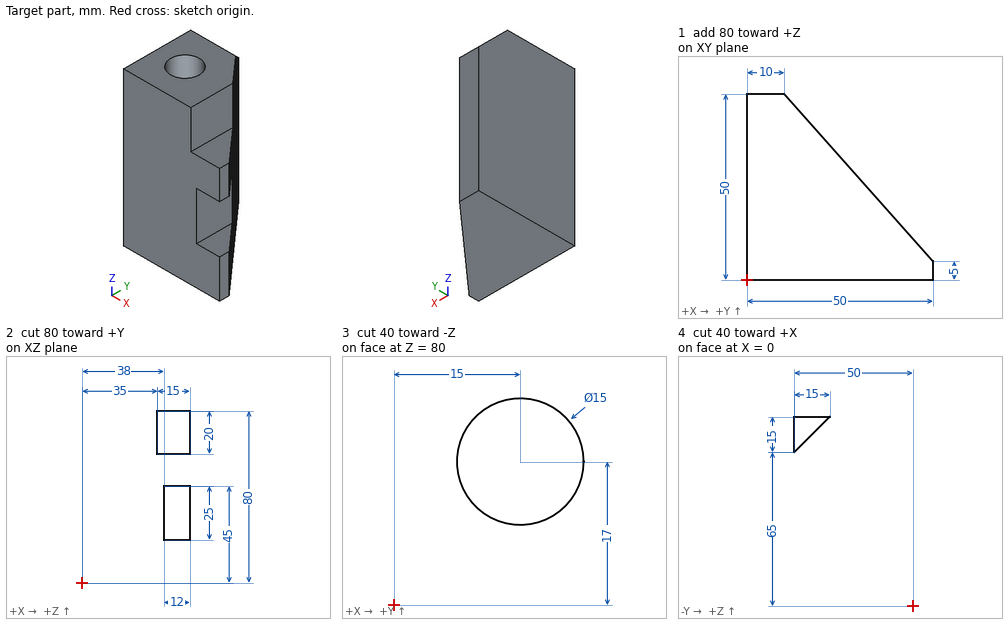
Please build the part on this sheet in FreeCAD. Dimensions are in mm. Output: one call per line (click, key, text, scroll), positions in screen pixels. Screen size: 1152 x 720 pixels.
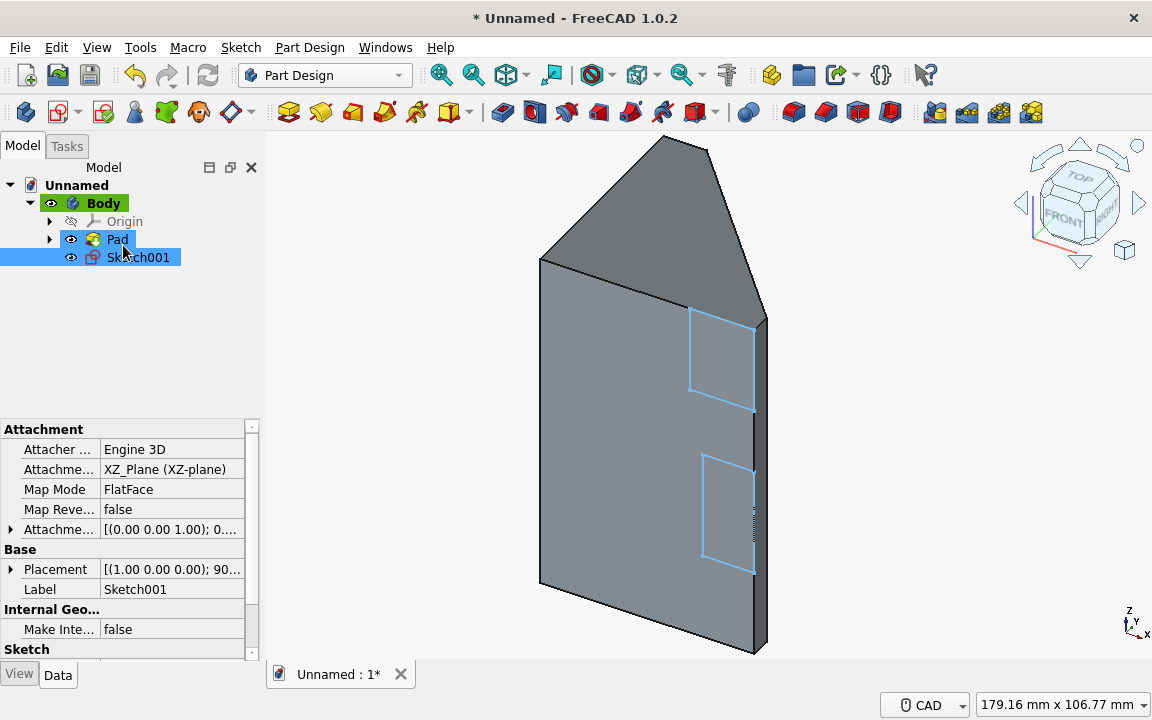
click(504, 112)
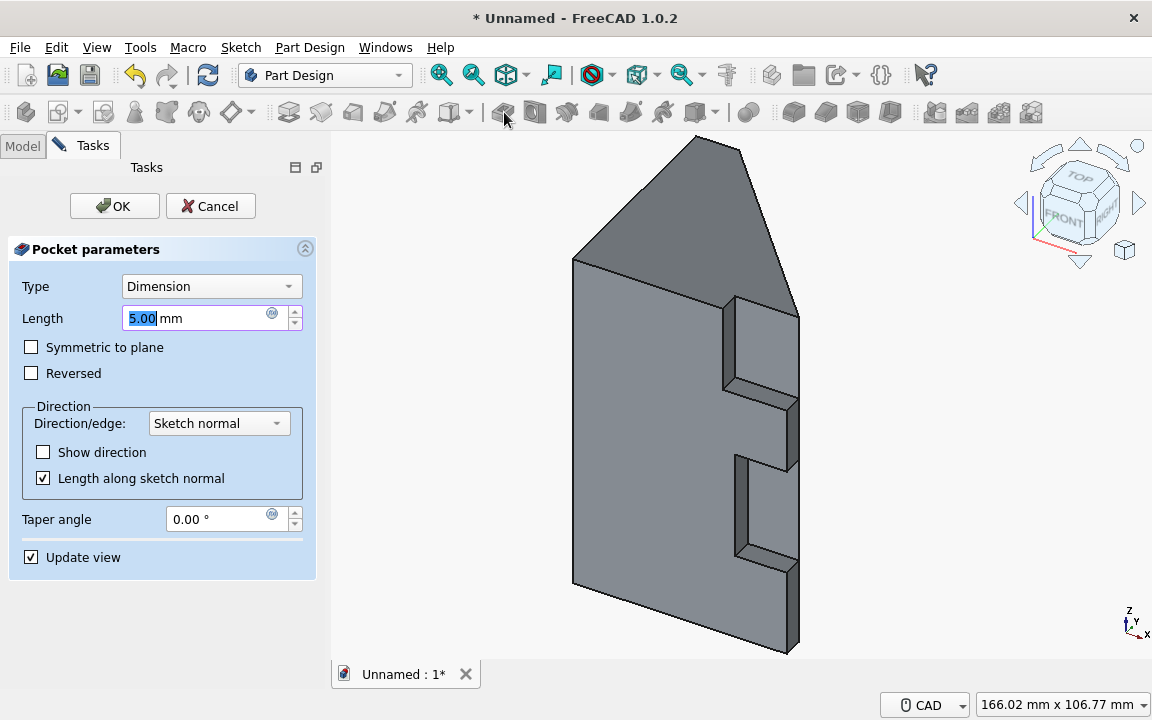
text(80)
key(Tab)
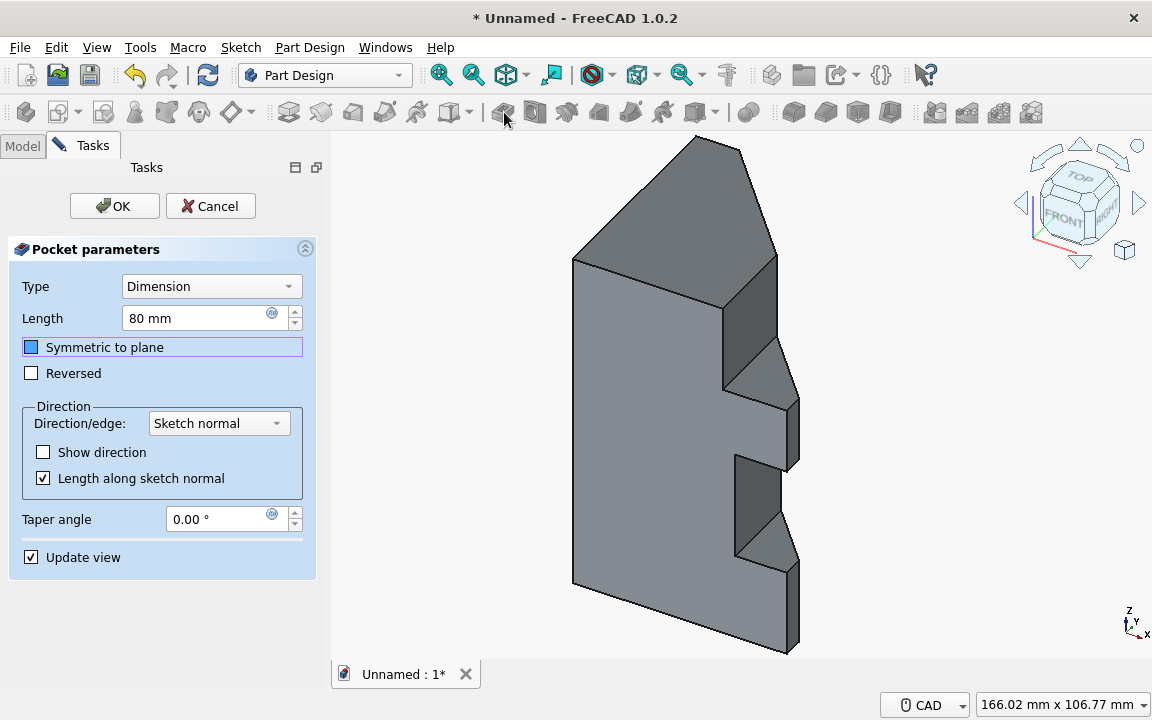
click(115, 206)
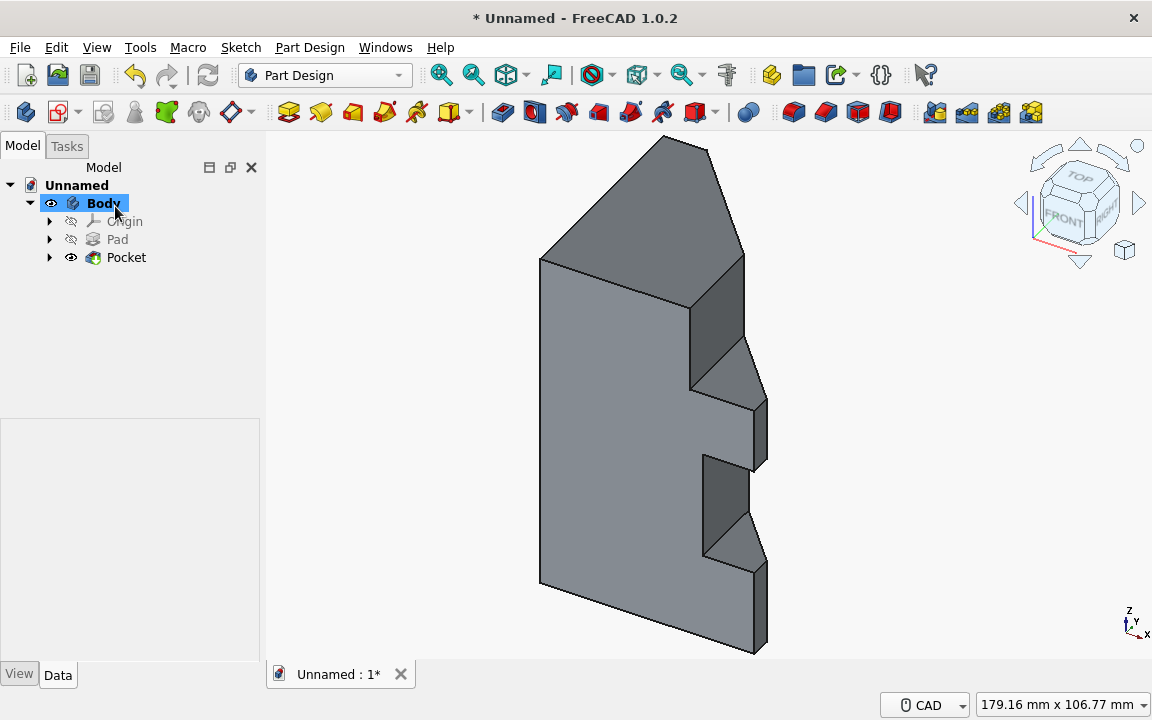
click(659, 239)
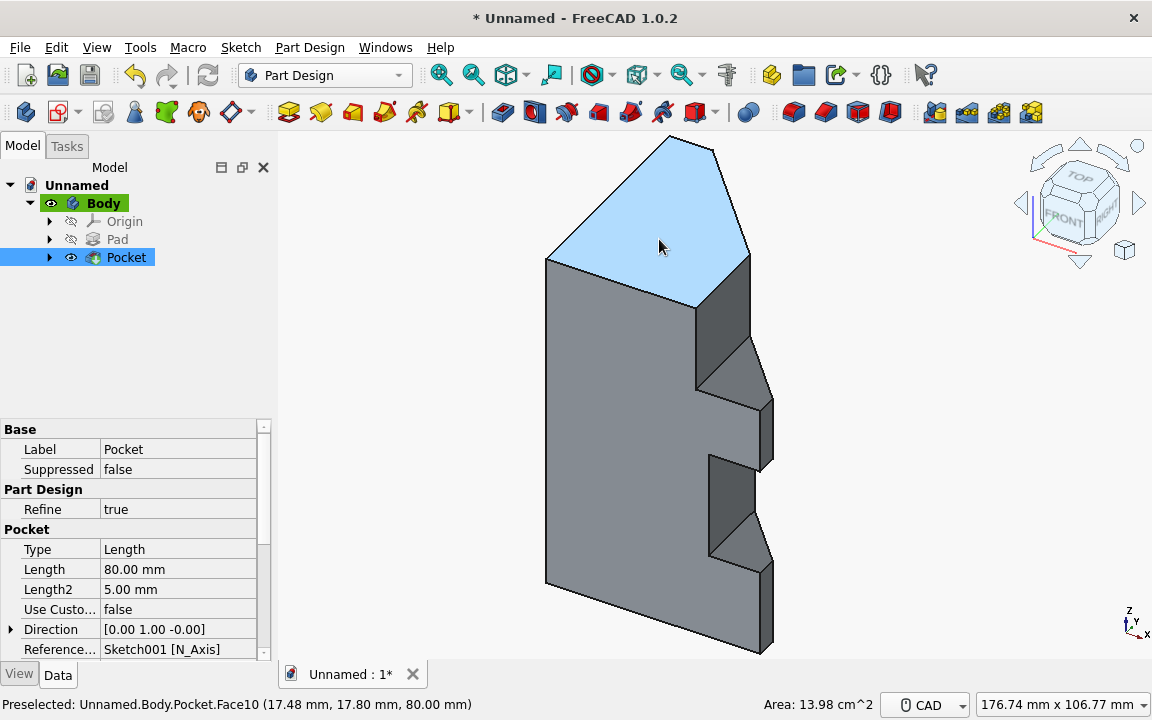
click(58, 112)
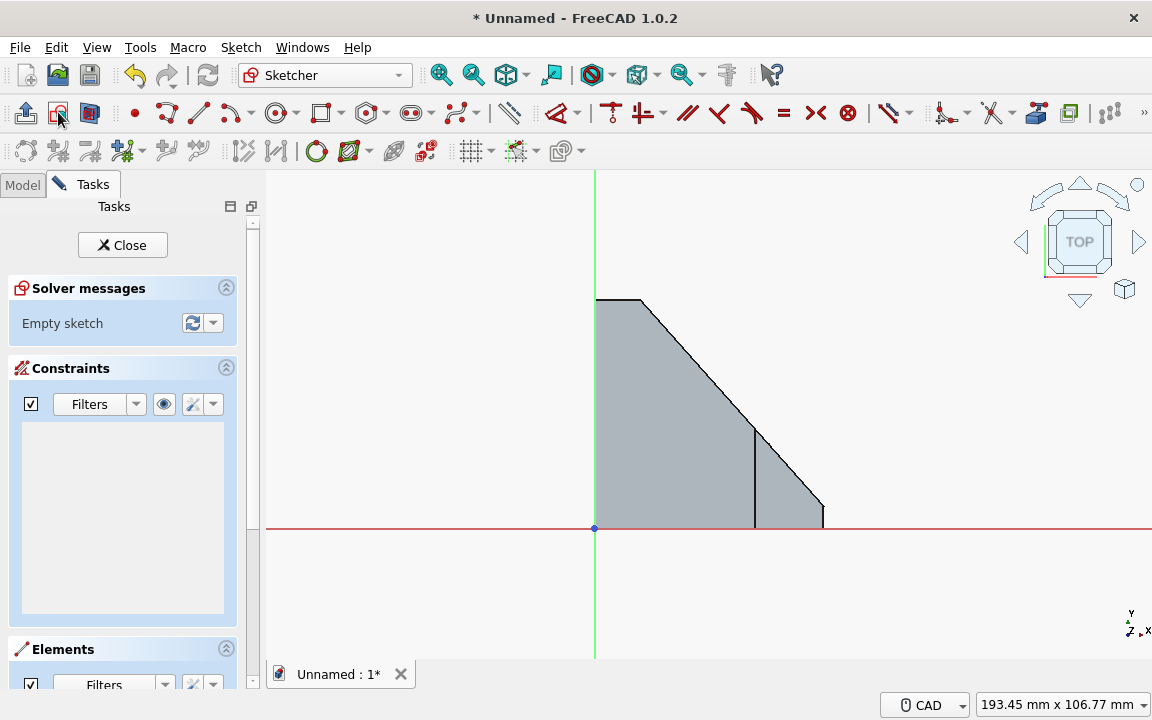
scroll(649, 507, up, 5)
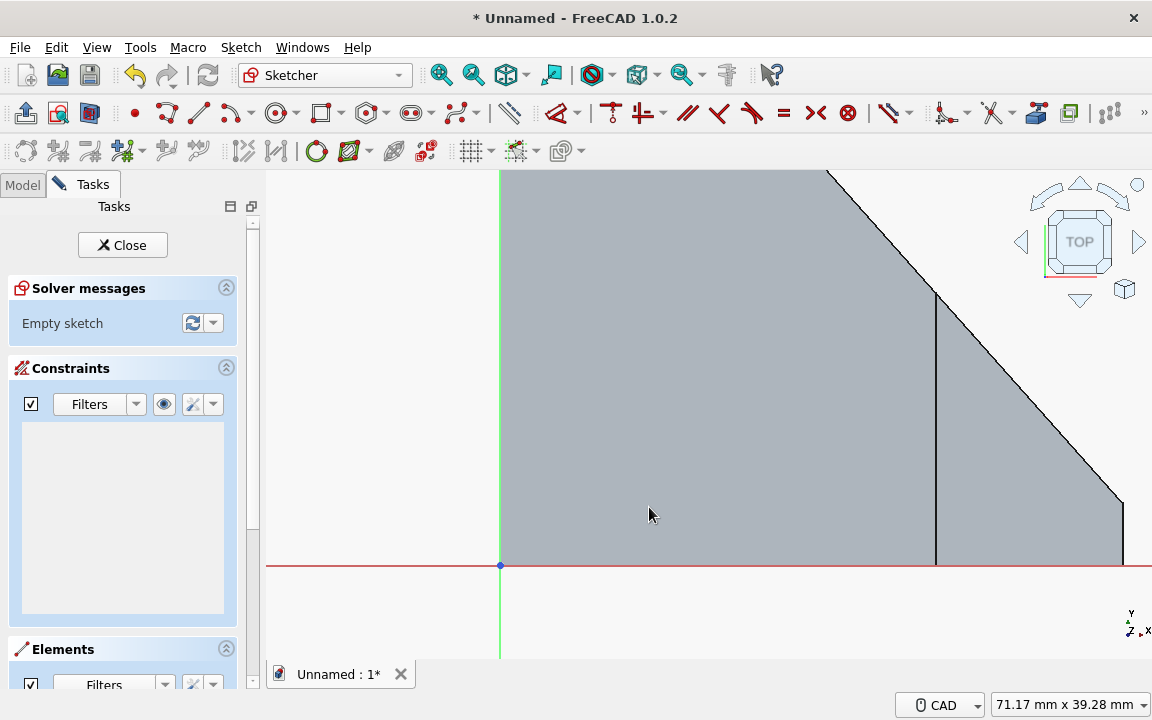
click(276, 114)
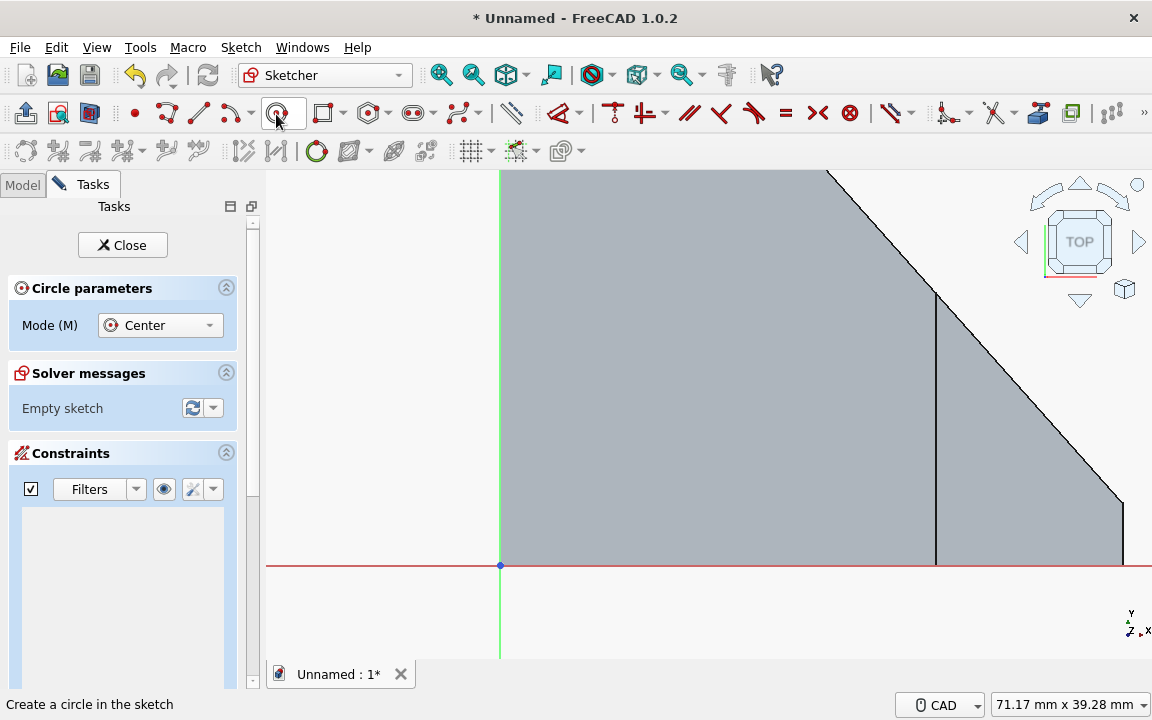
click(687, 354)
click(753, 288)
key(Escape)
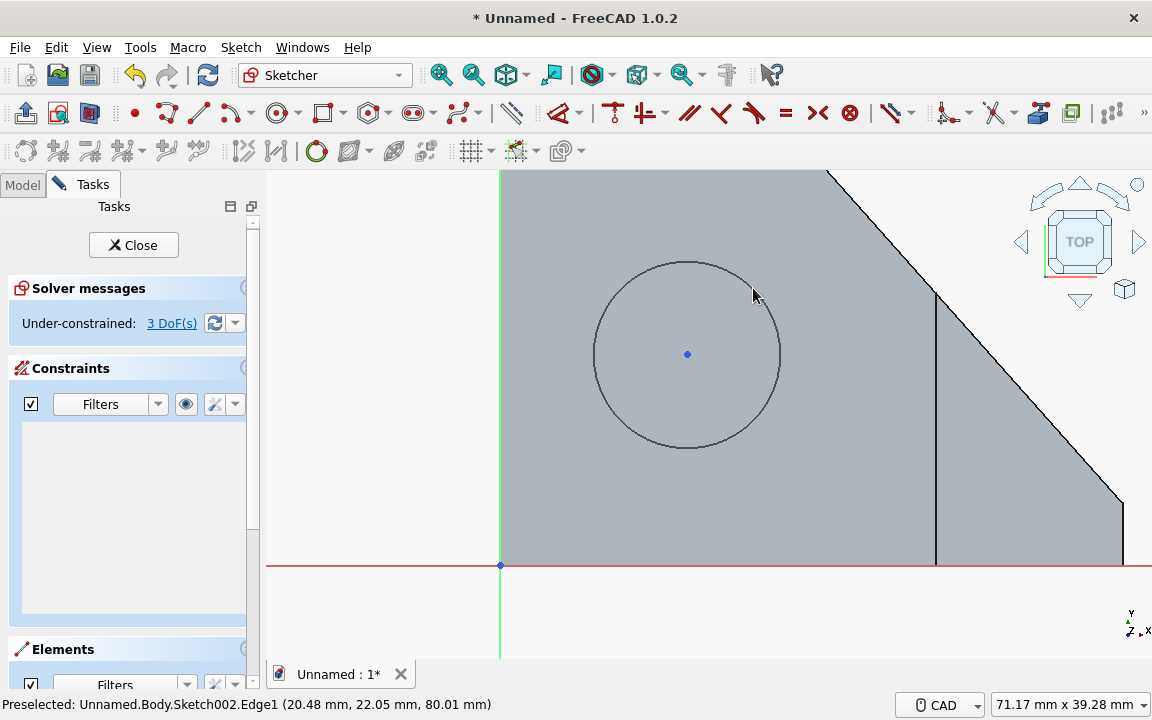
click(558, 114)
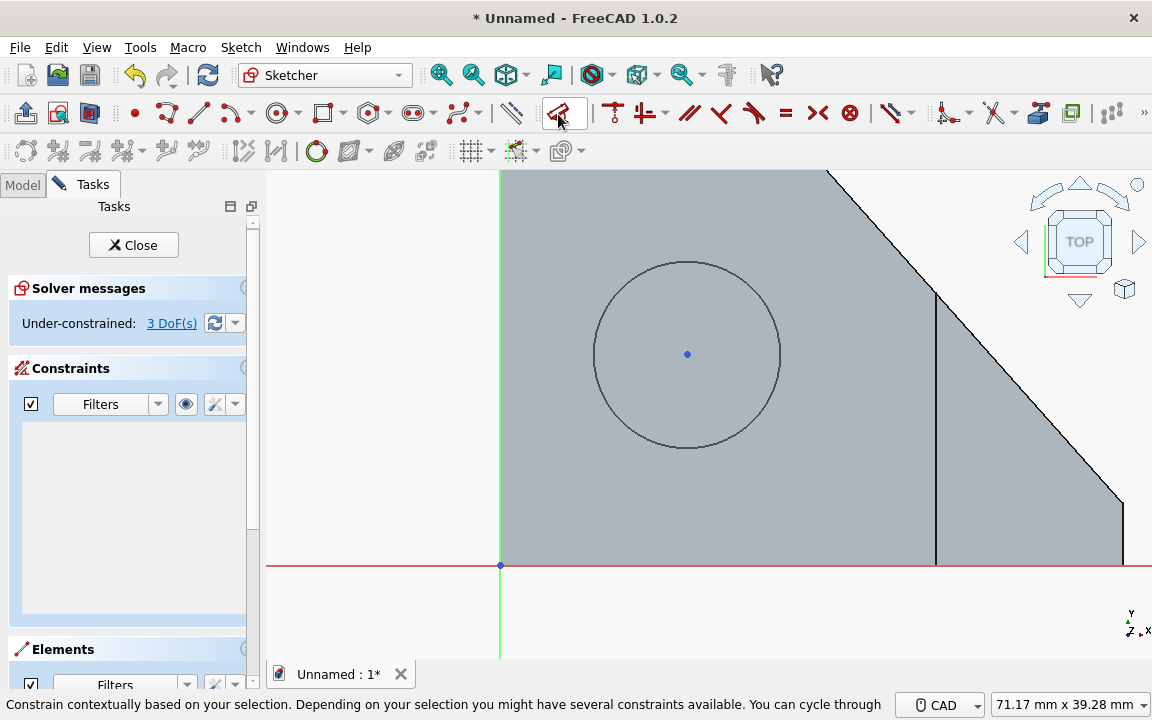
click(753, 289)
click(776, 266)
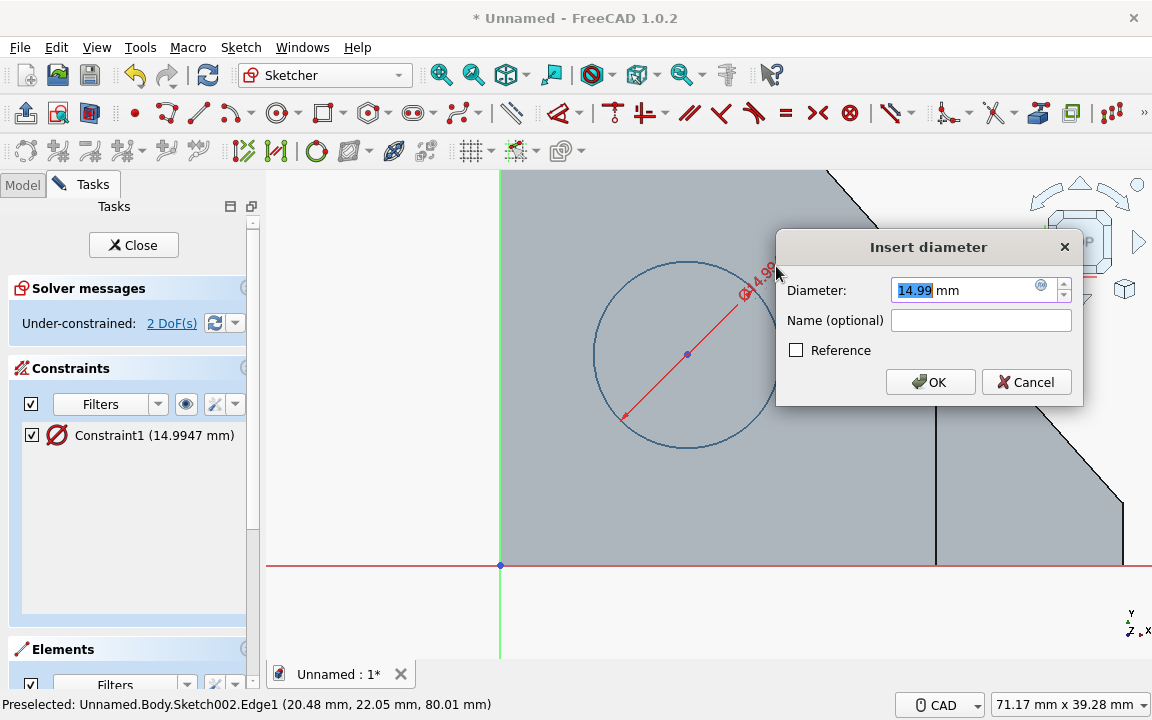
text(15)
key(Return)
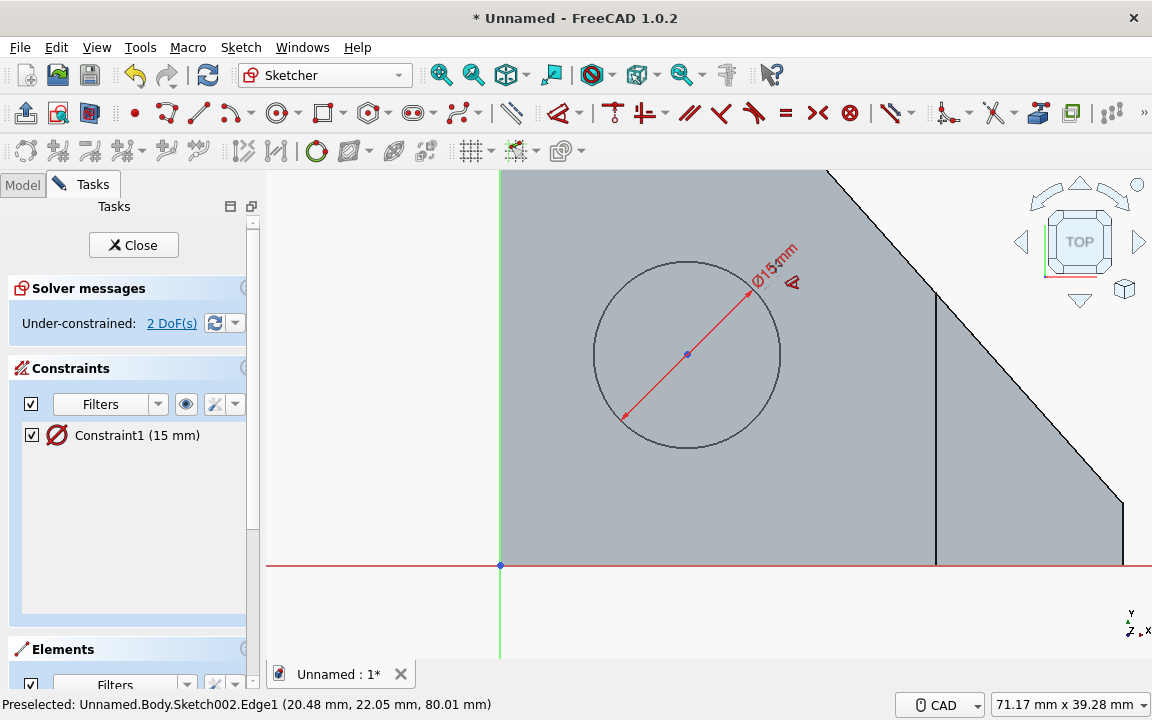
click(687, 355)
click(594, 600)